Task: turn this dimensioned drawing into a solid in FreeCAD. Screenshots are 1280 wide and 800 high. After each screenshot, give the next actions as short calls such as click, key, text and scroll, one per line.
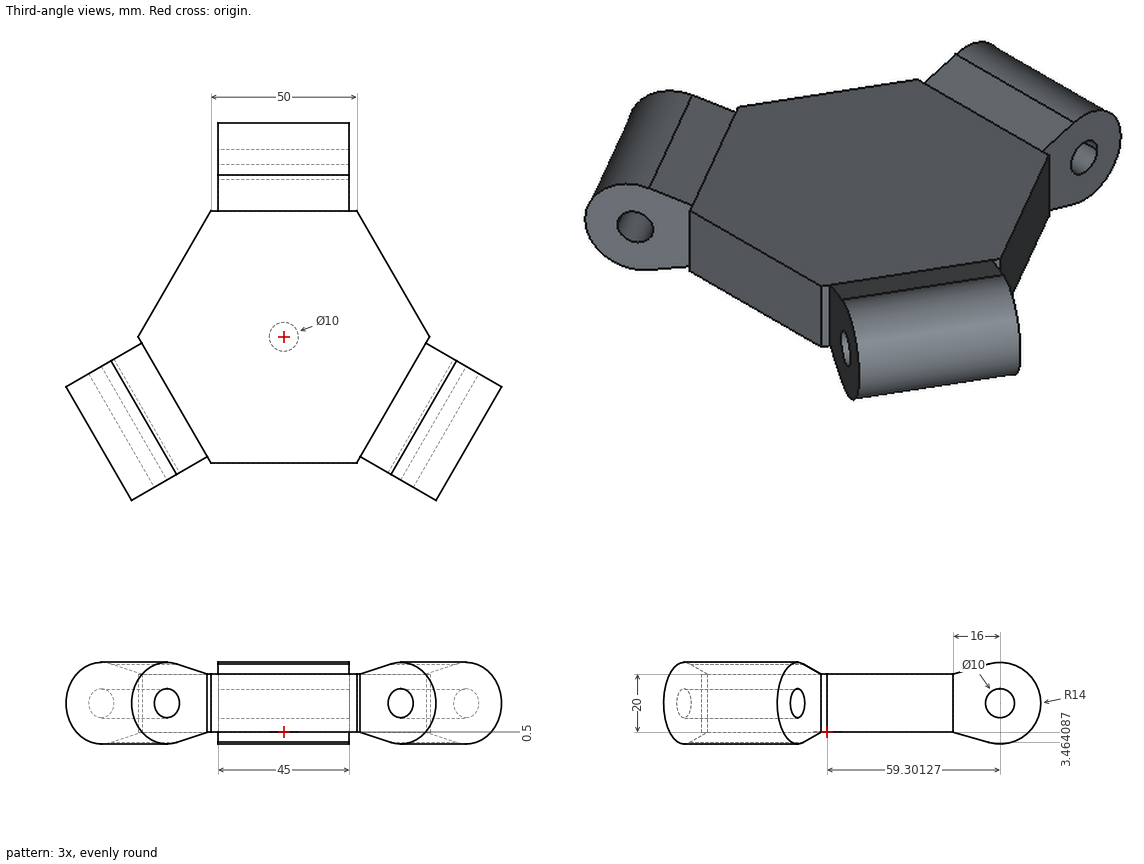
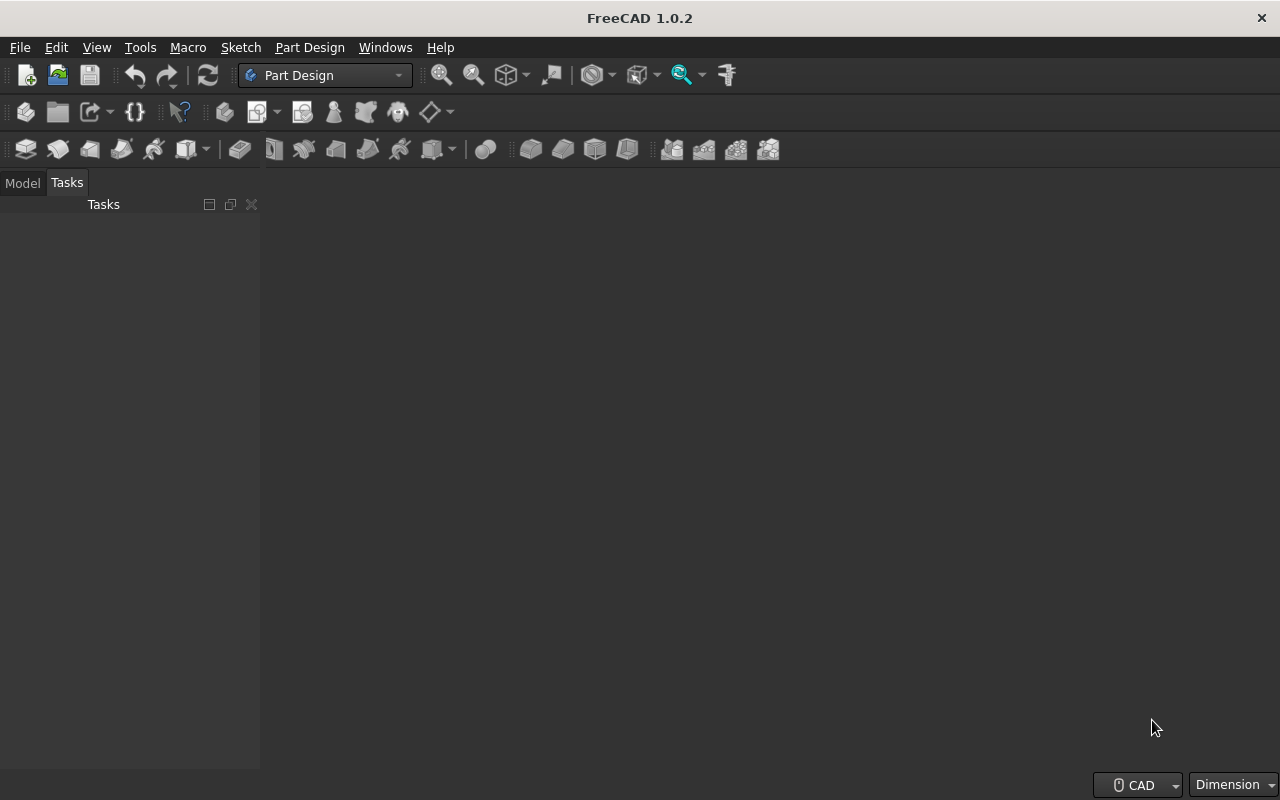
click(26, 76)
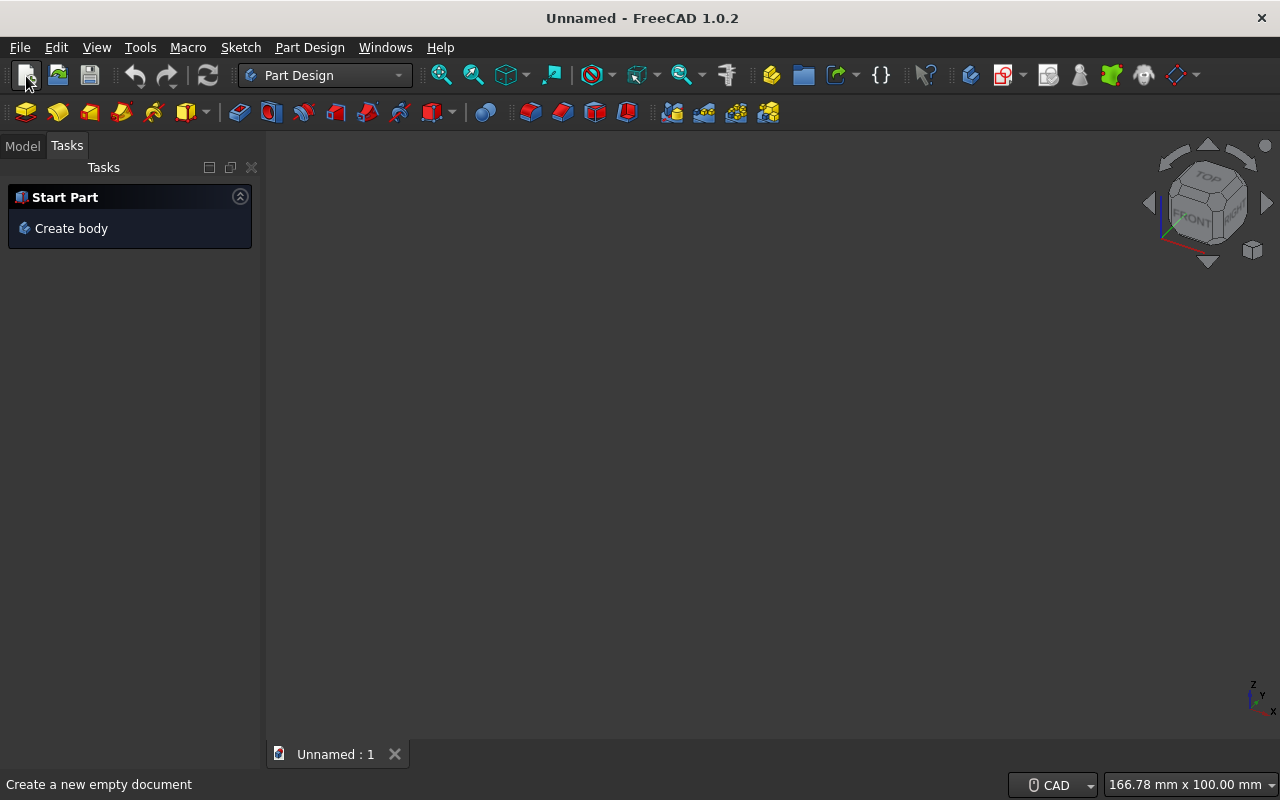
click(1004, 76)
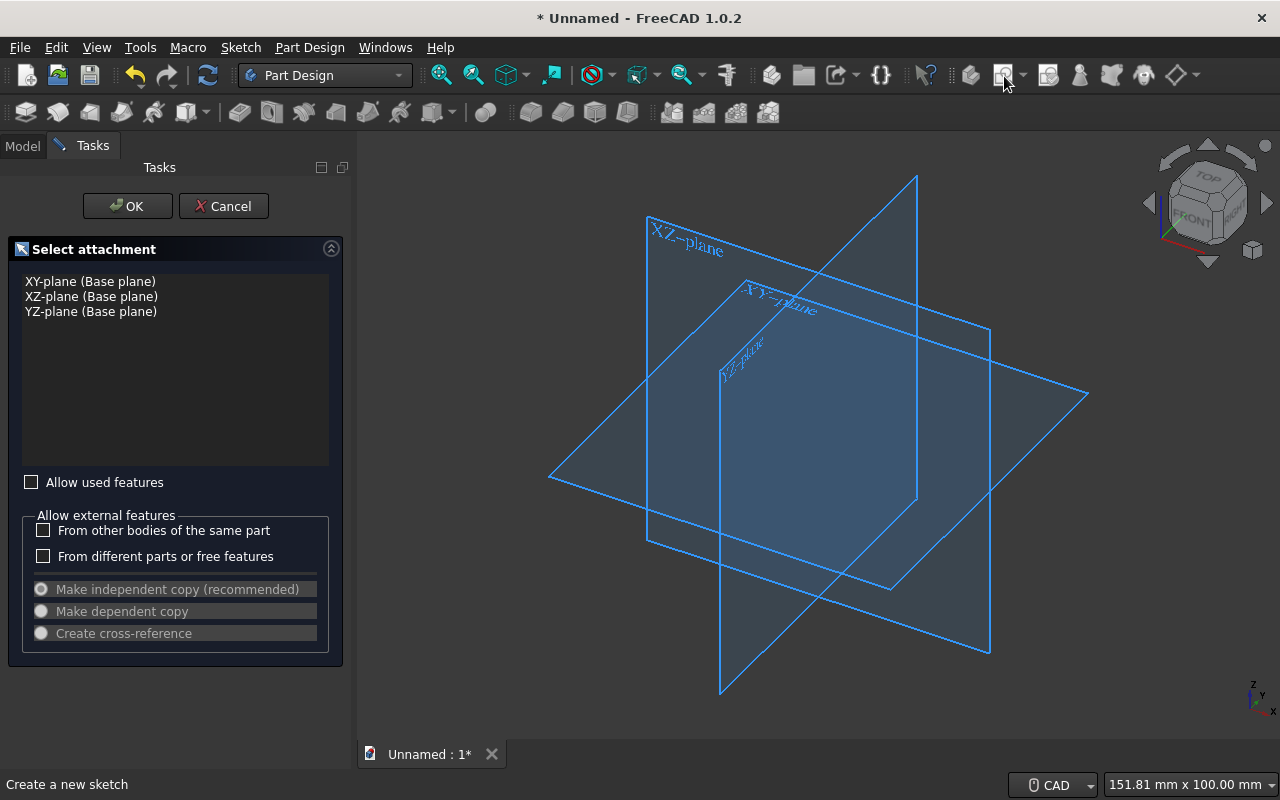
click(82, 282)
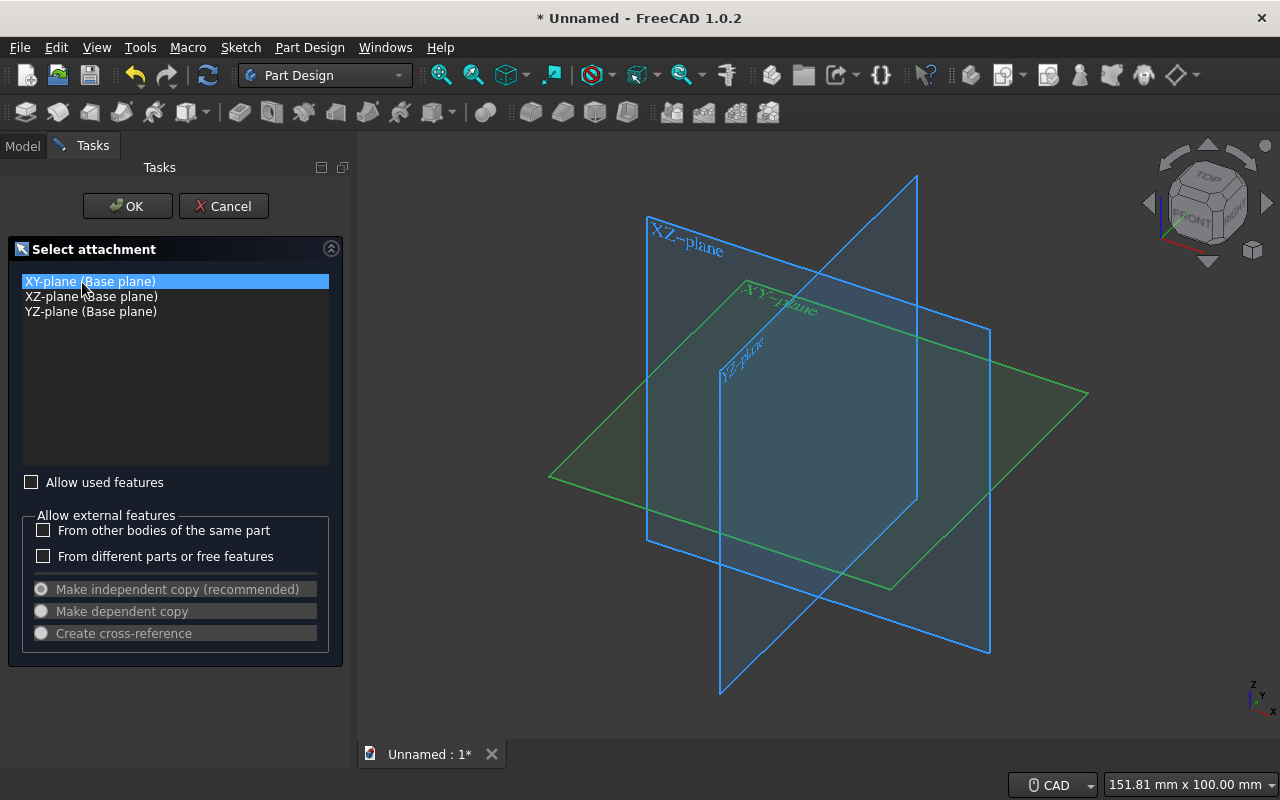
click(128, 206)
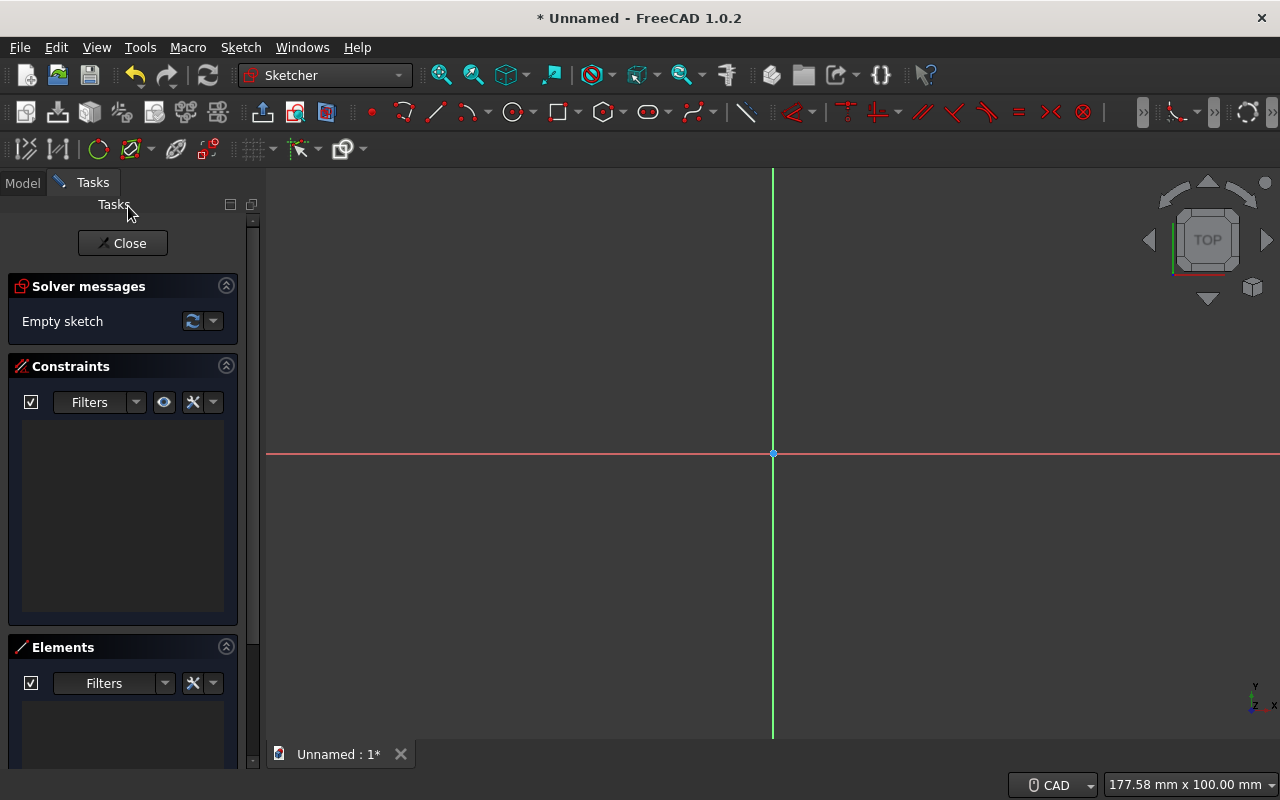
scroll(565, 453, down, 2)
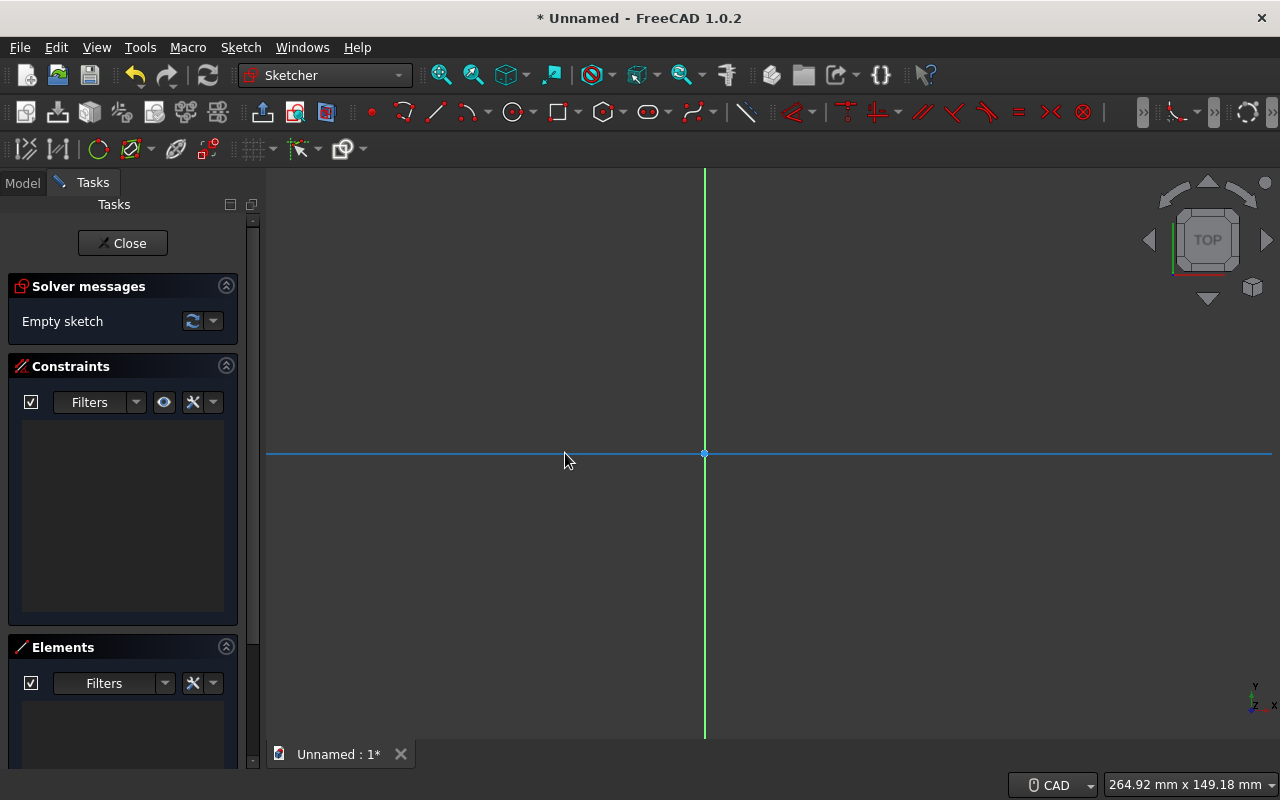
click(604, 112)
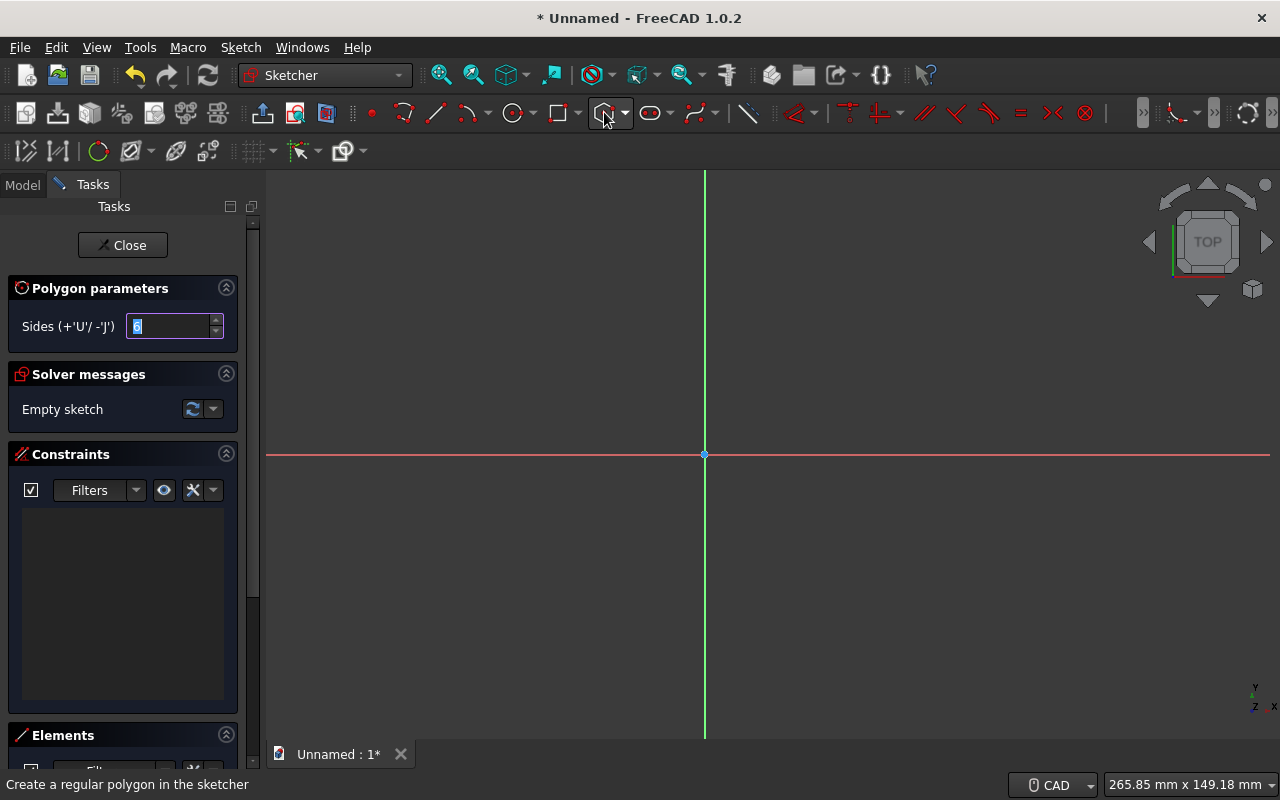
click(705, 454)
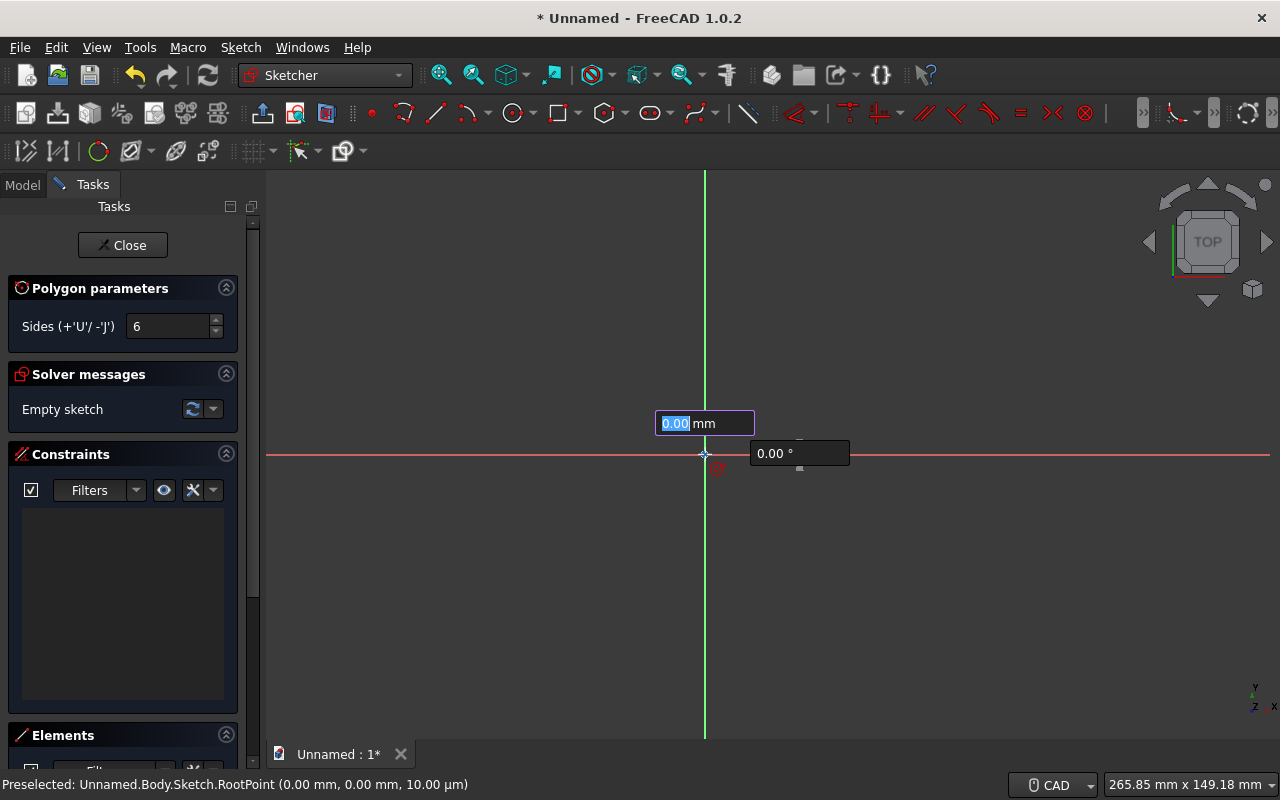
click(895, 454)
right_click(895, 454)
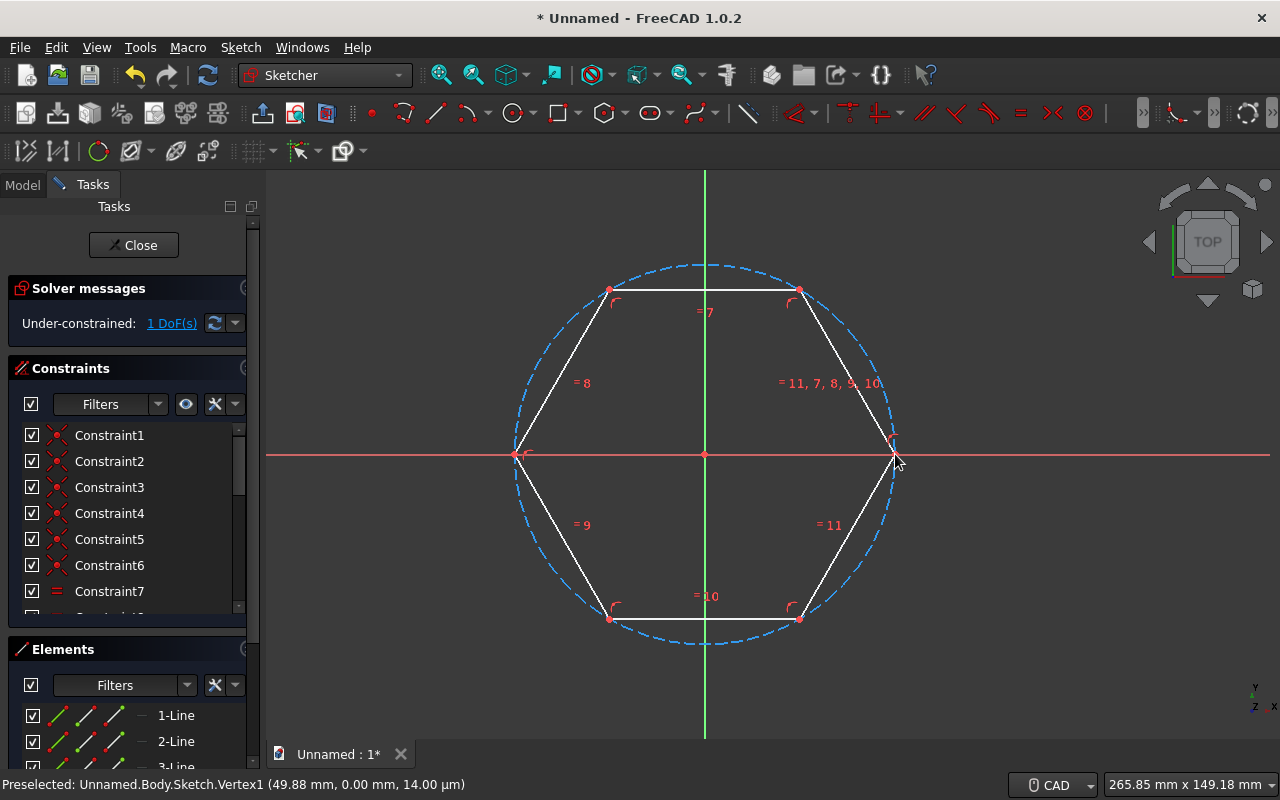
click(794, 114)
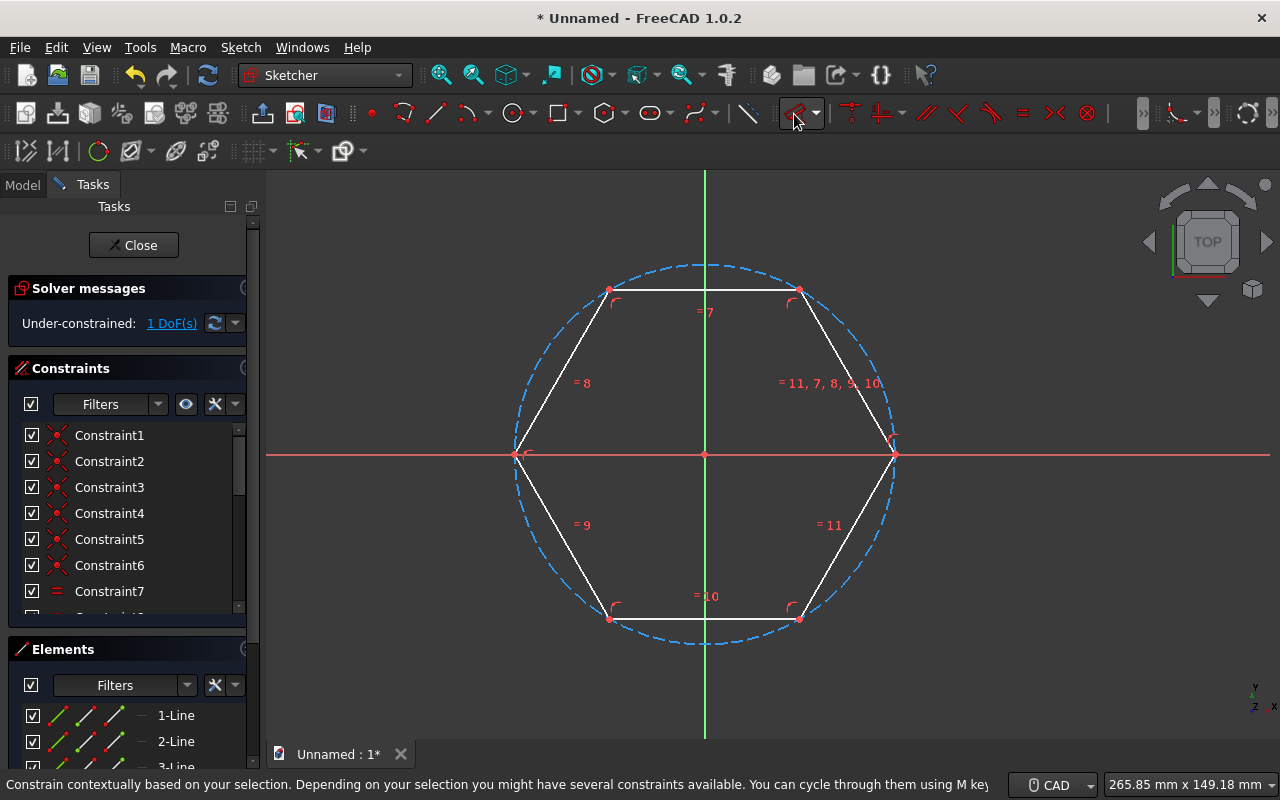
click(743, 290)
click(661, 256)